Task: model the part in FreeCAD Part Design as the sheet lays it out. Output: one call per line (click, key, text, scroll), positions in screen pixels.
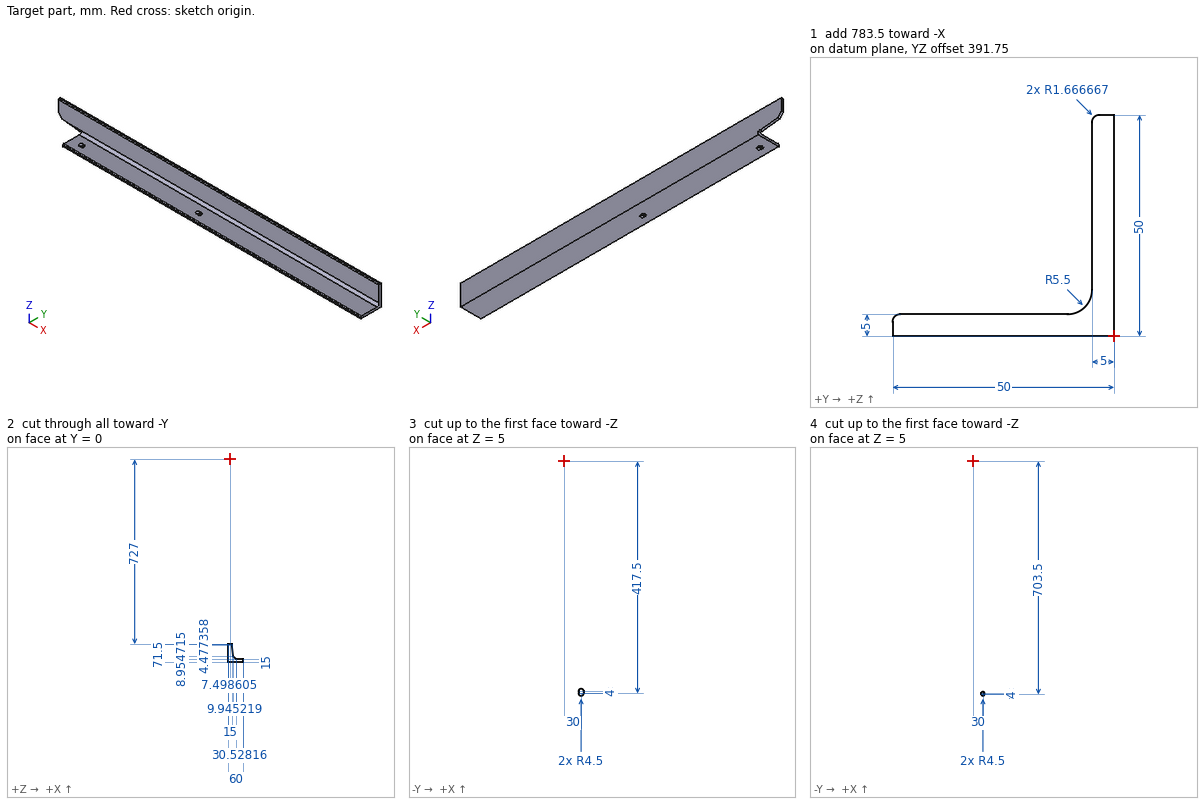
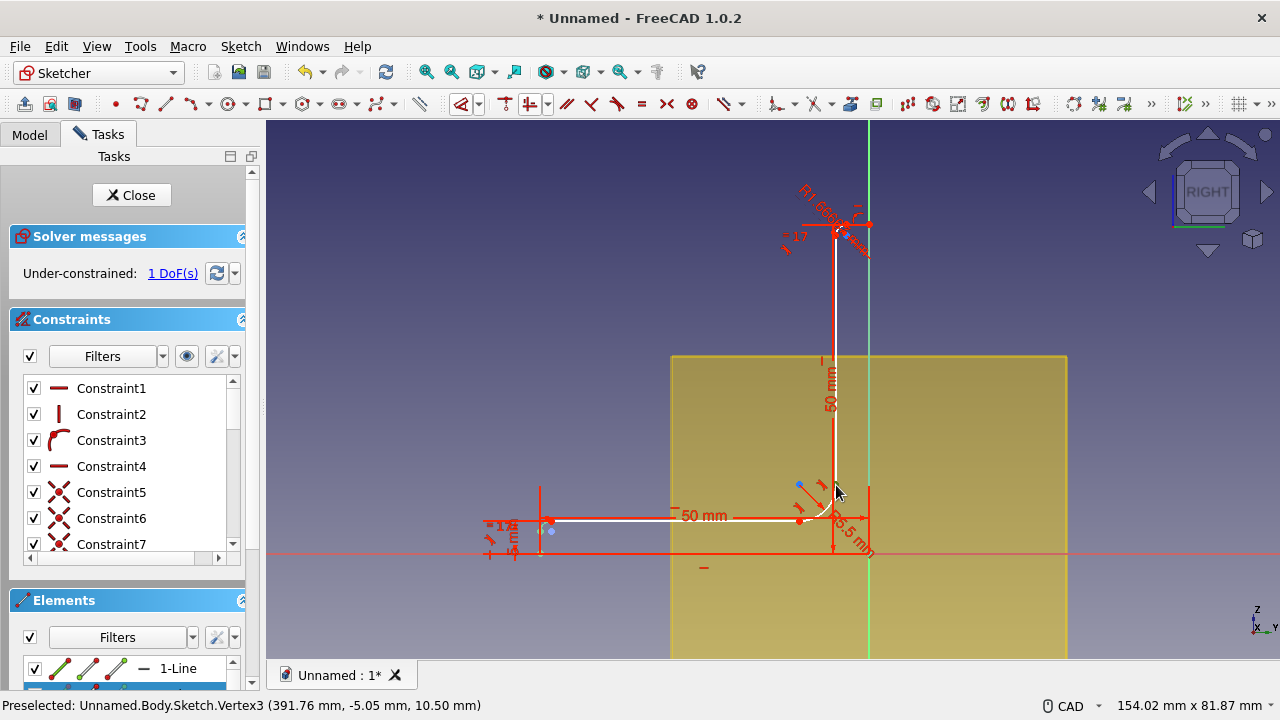
click(478, 104)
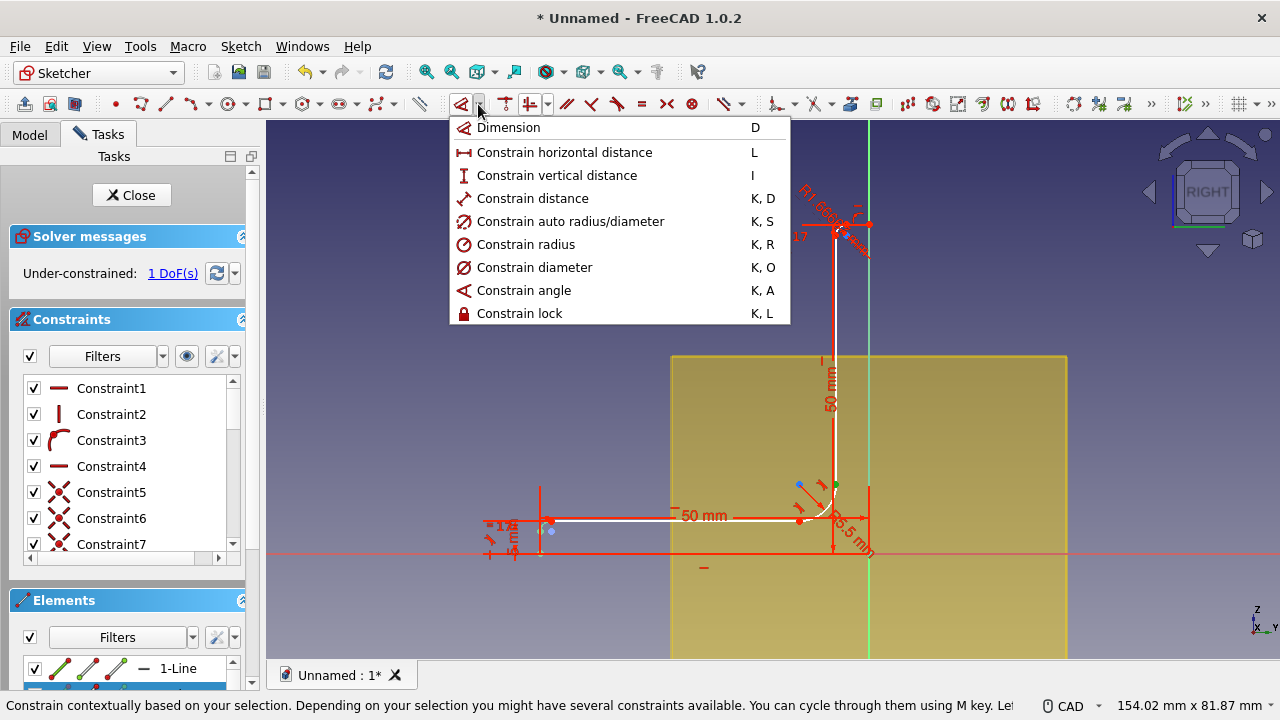
click(620, 152)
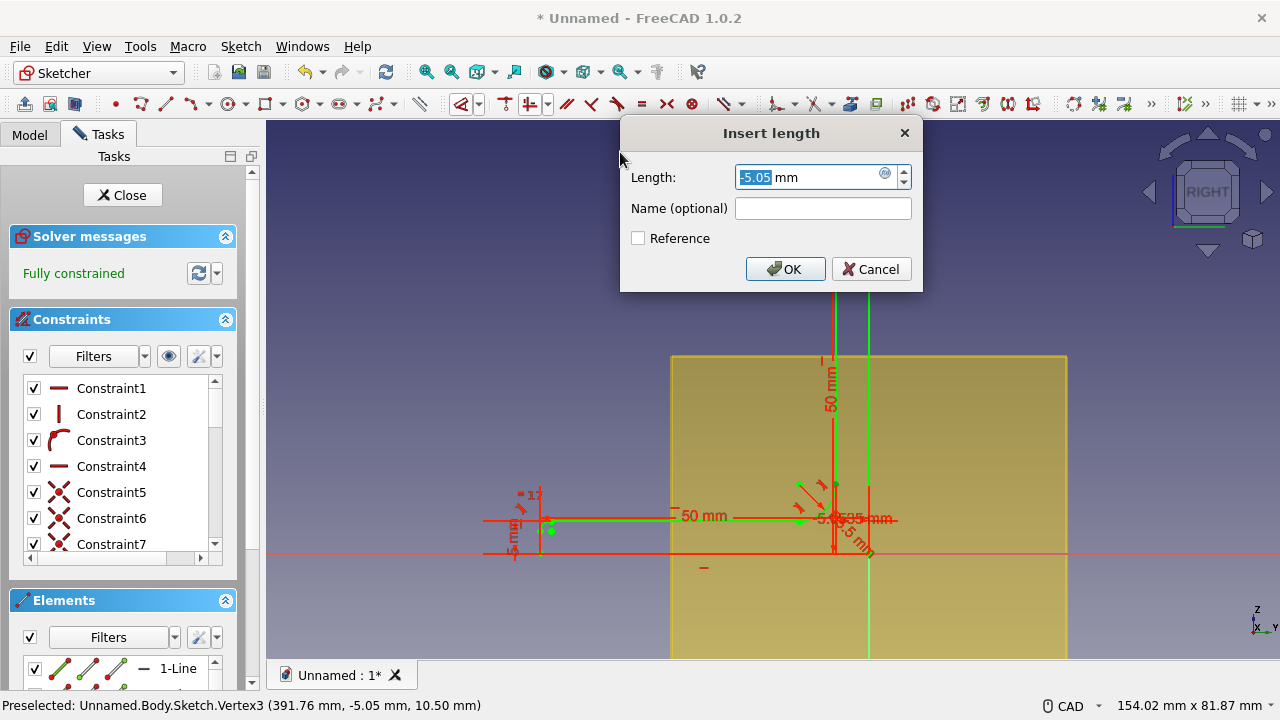
text(-5)
key(Return)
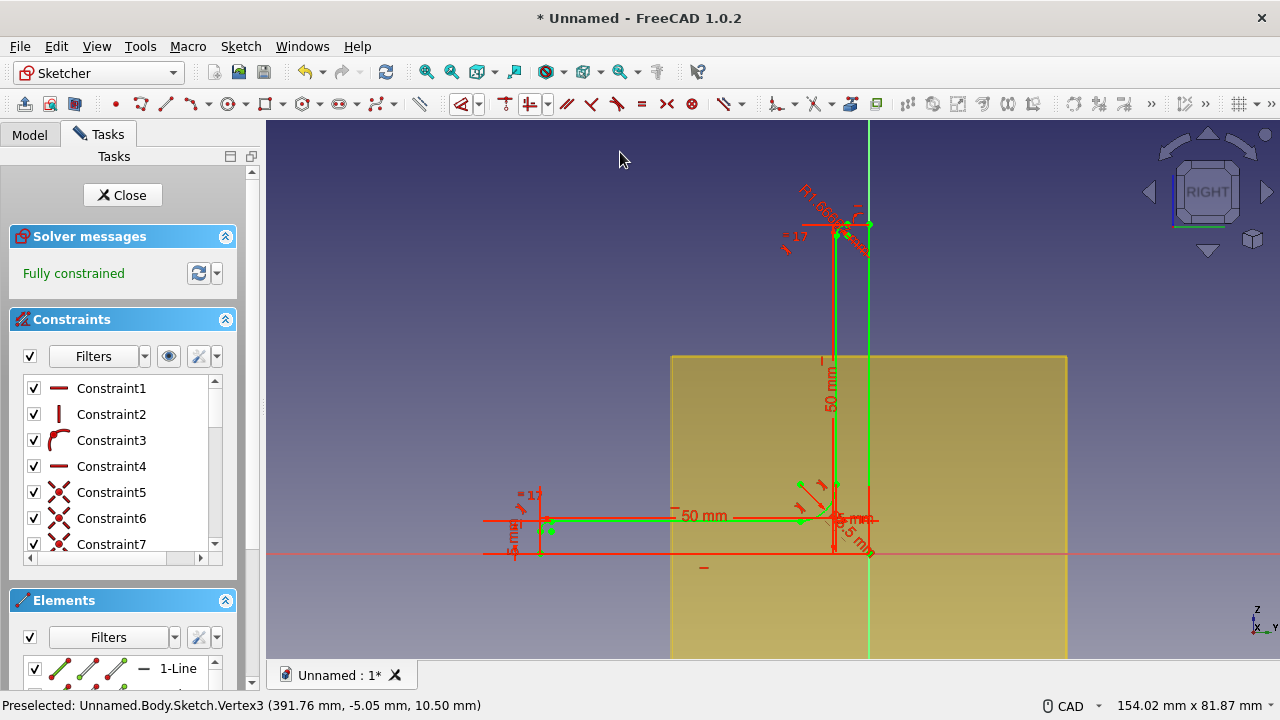
click(123, 195)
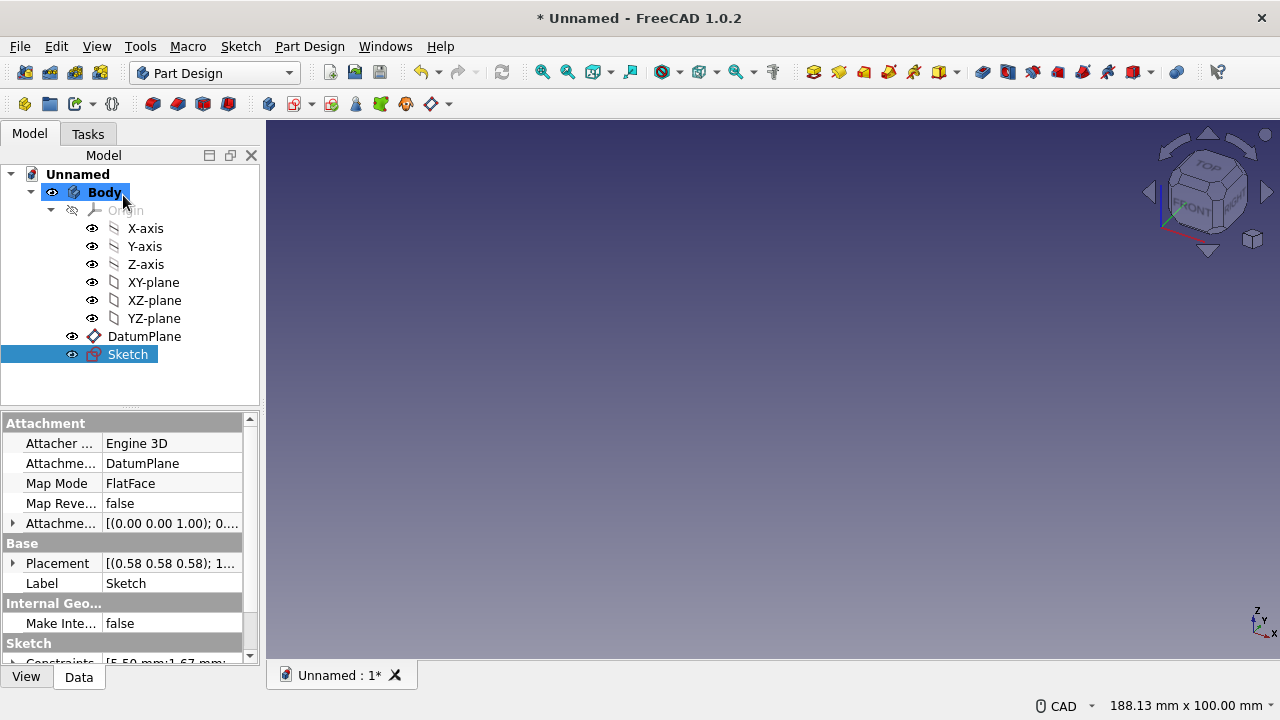
click(814, 72)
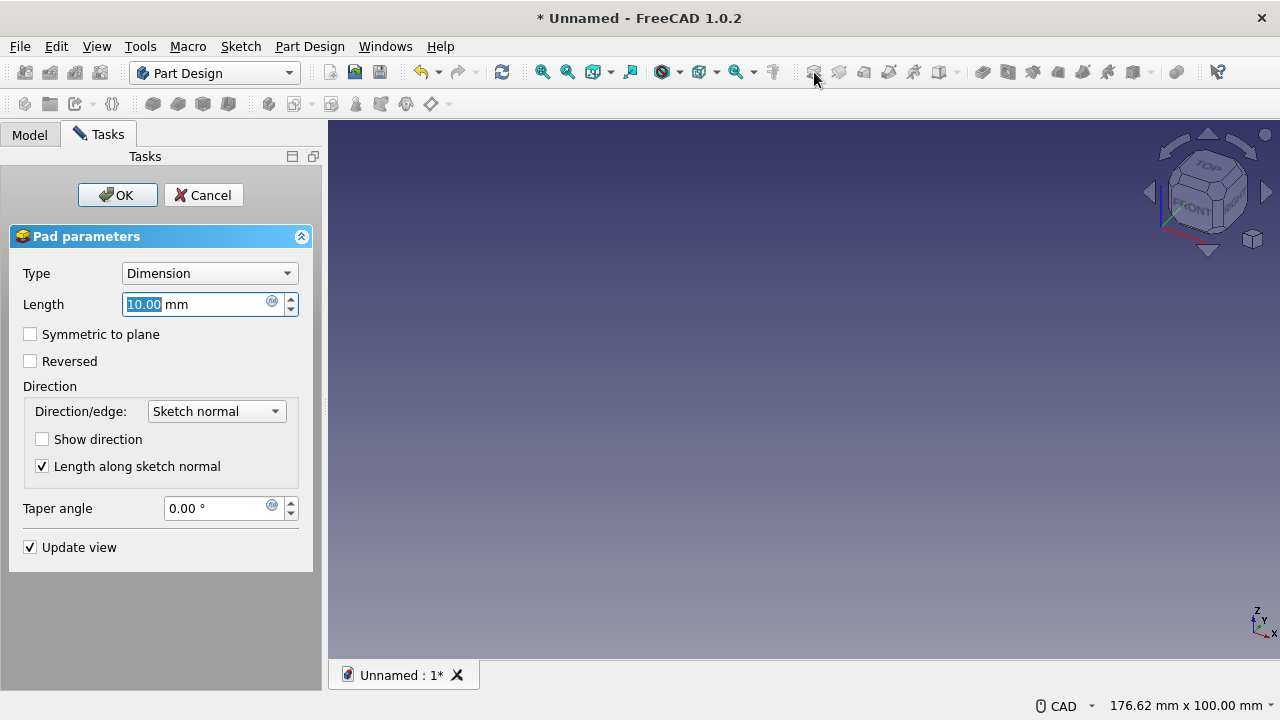
text(783.5)
key(Tab)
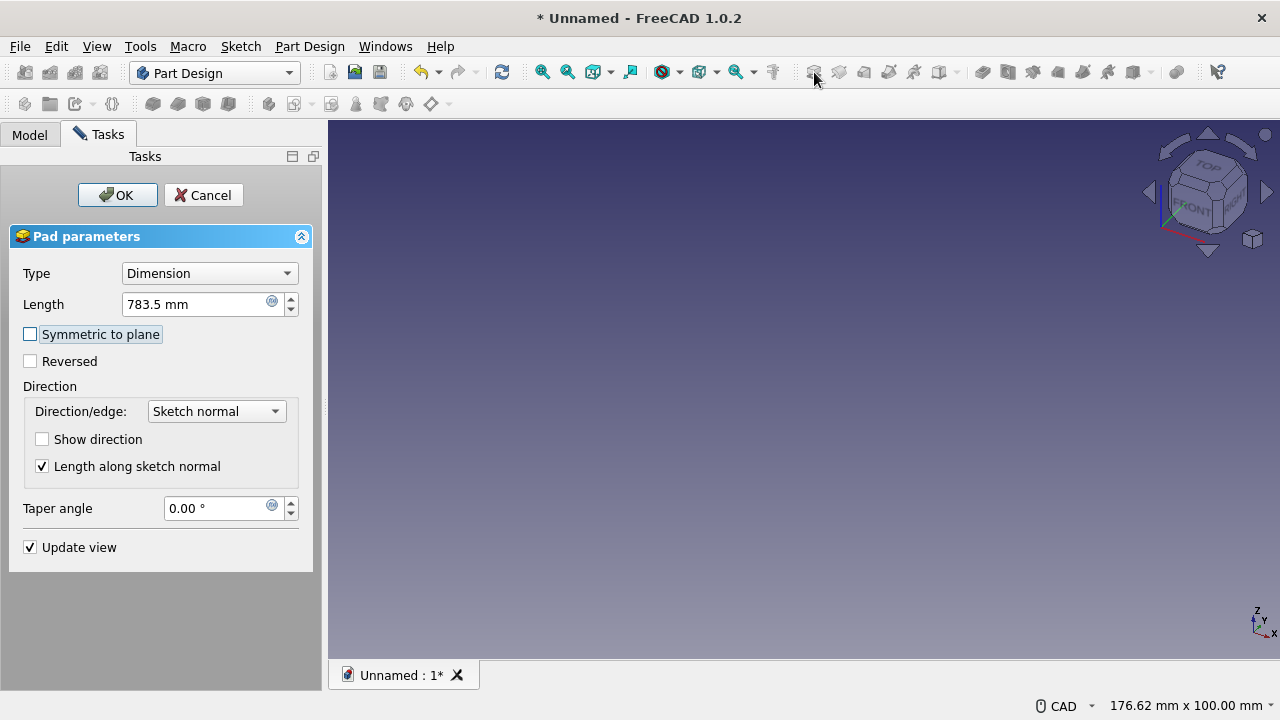
click(31, 361)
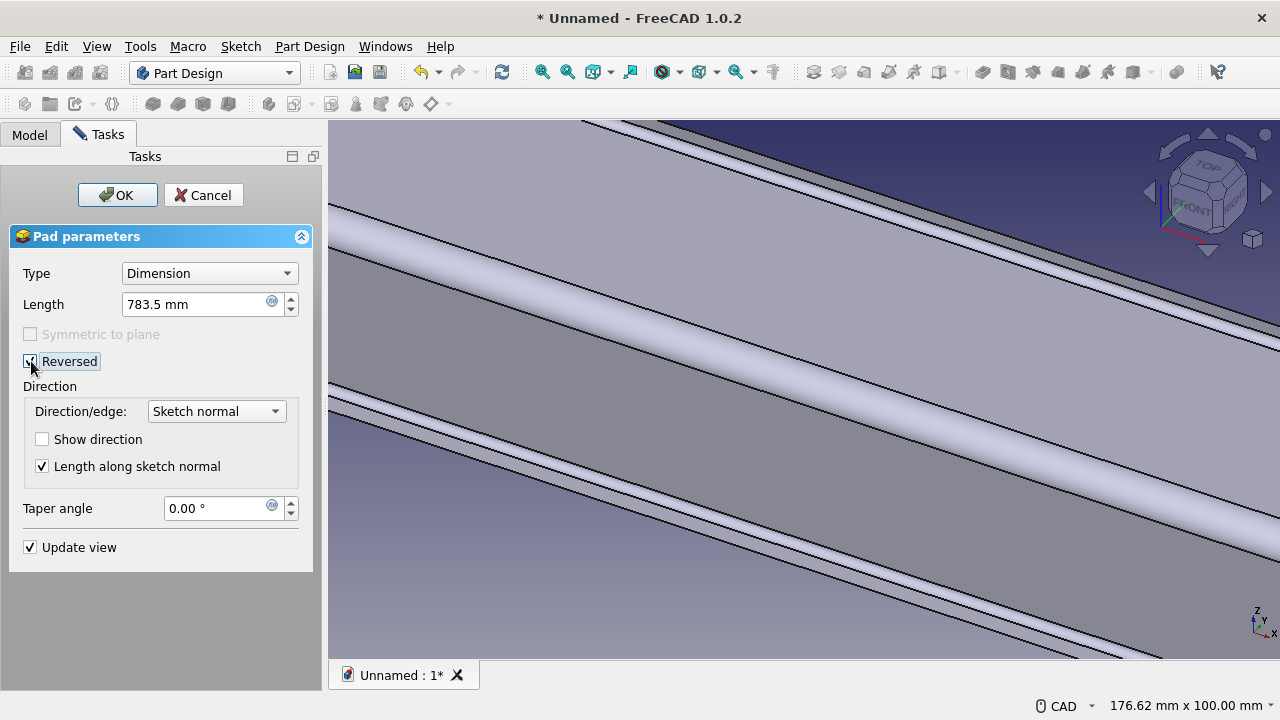
click(118, 195)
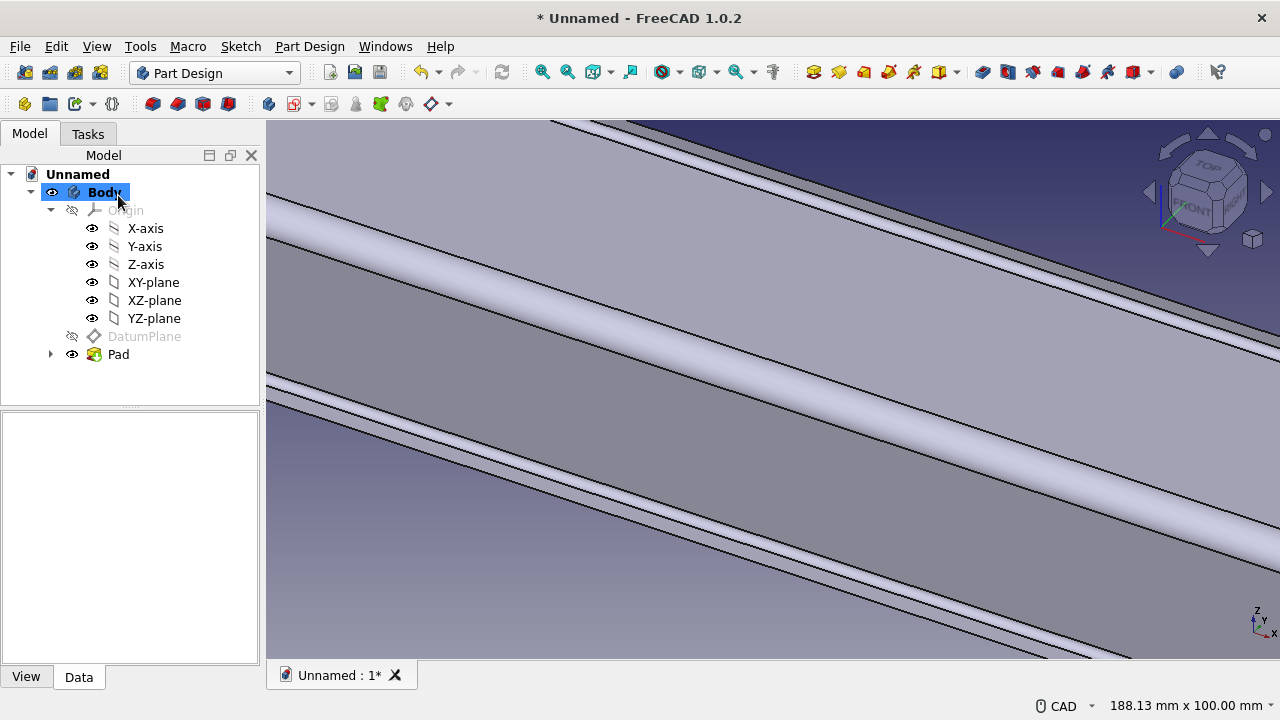
click(543, 72)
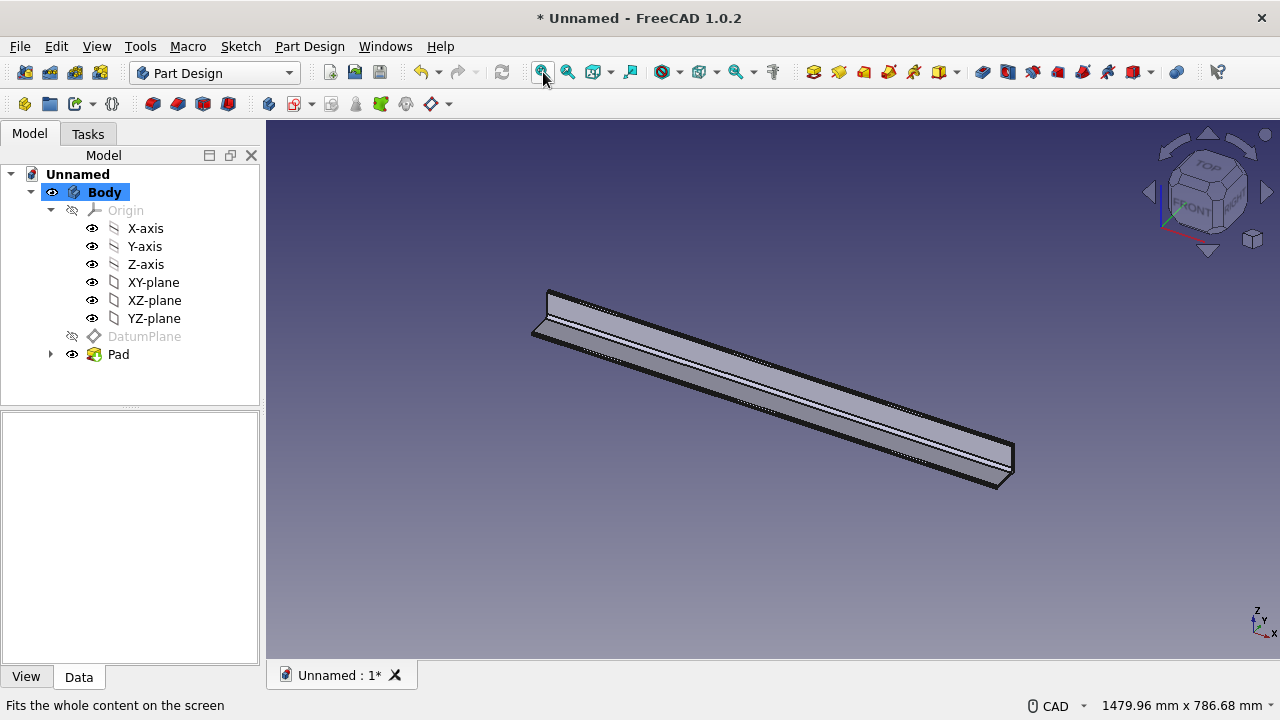
key(4)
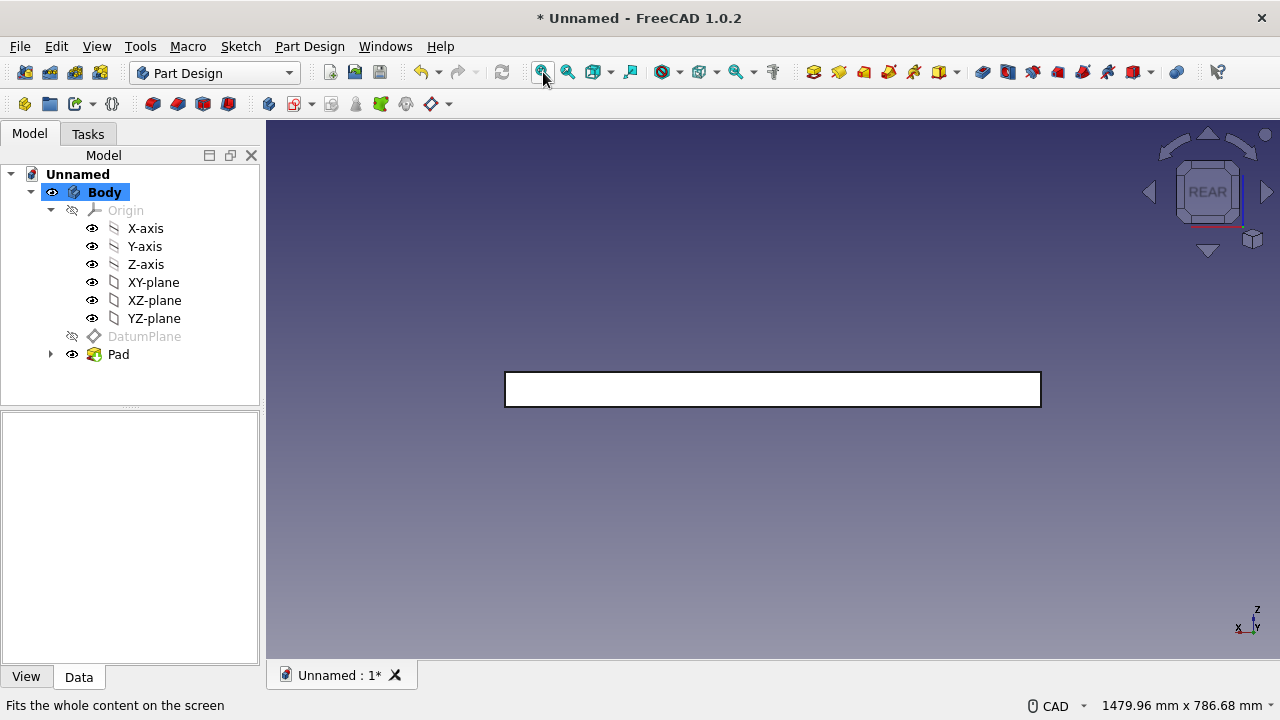
click(773, 388)